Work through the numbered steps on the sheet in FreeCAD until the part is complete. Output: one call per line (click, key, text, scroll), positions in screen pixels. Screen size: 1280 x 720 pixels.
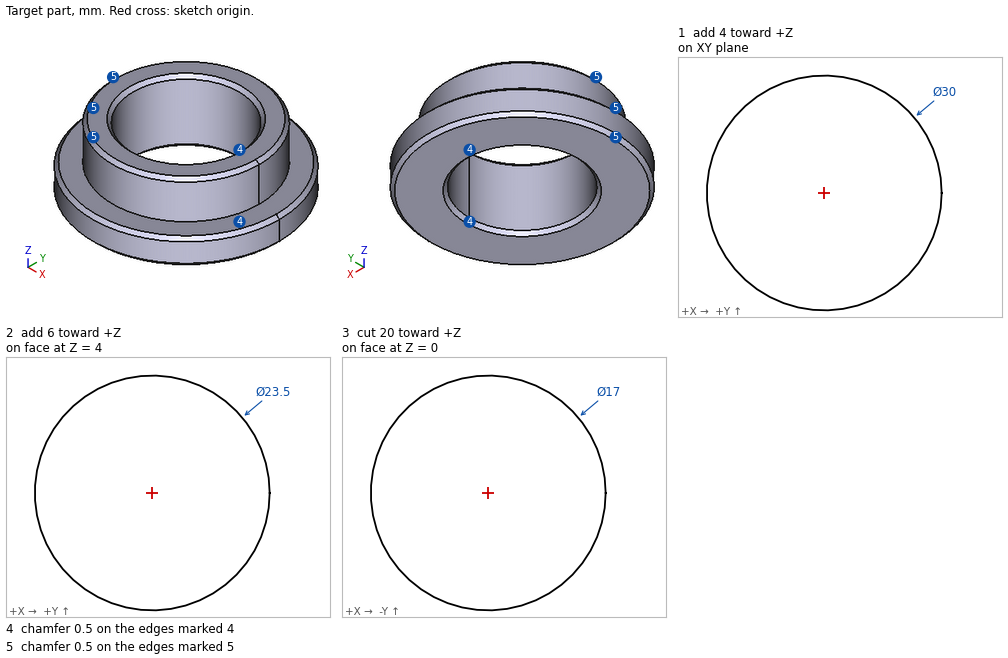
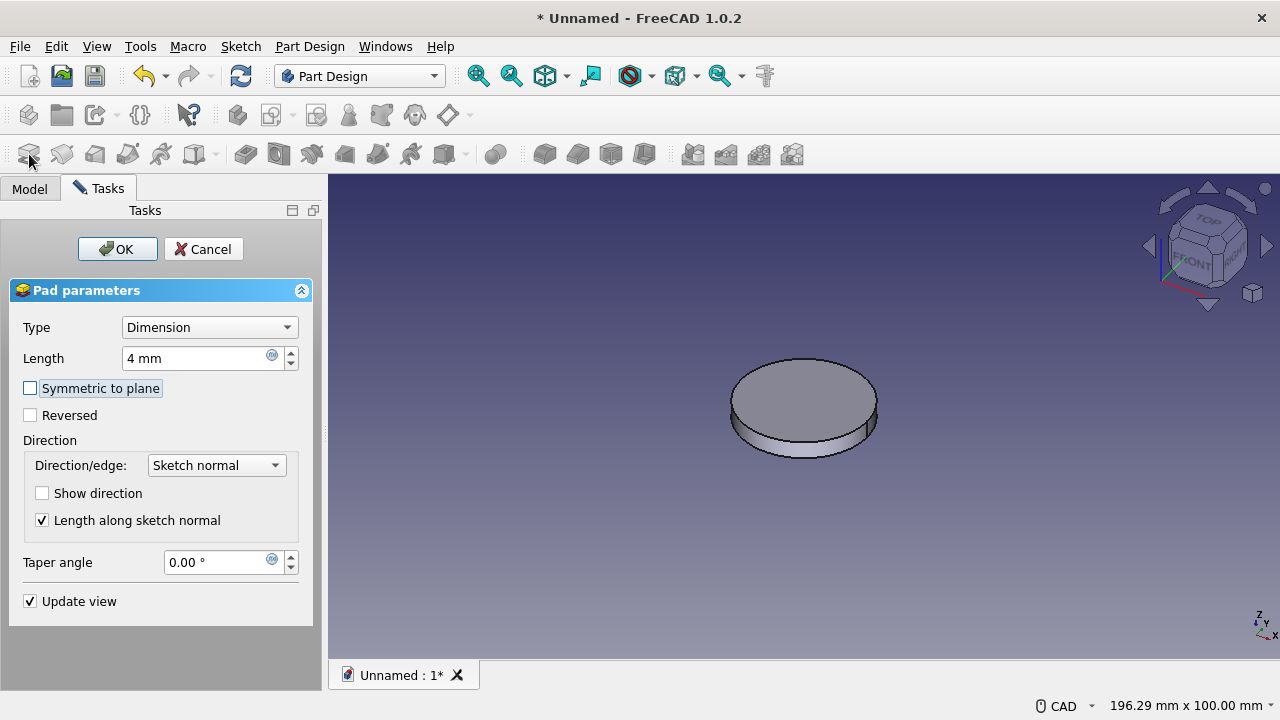
click(118, 249)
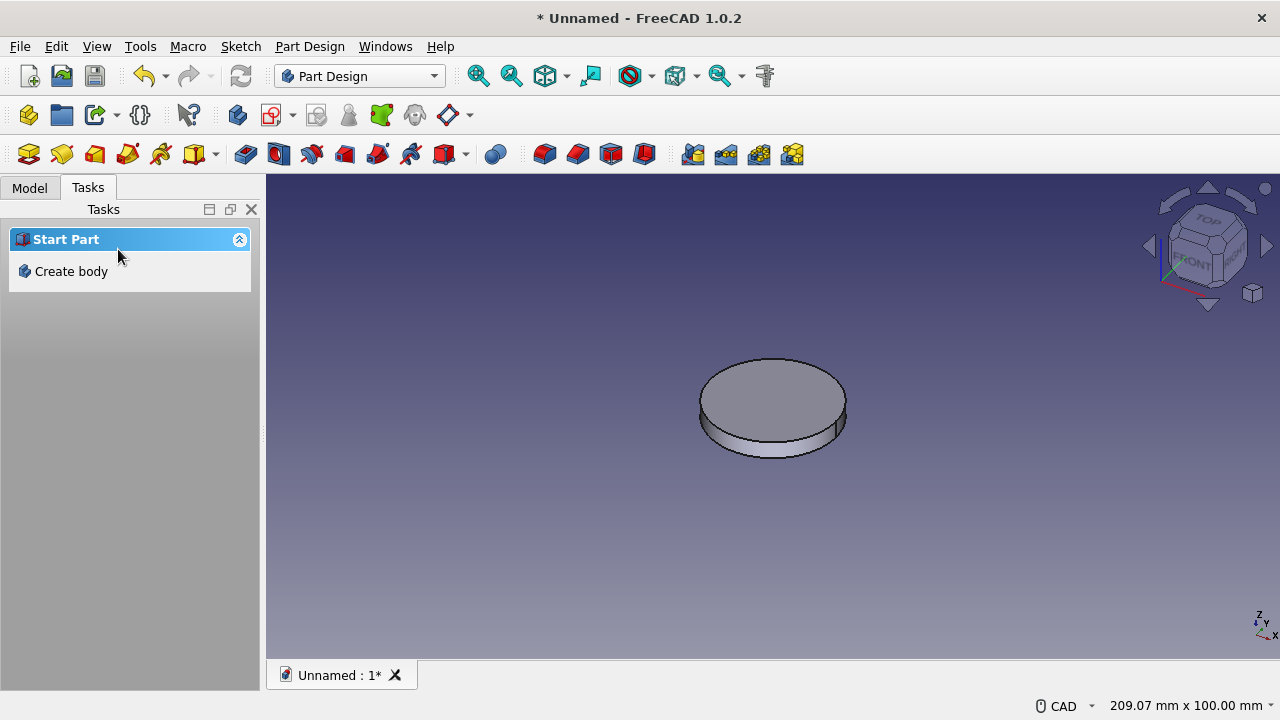
click(479, 76)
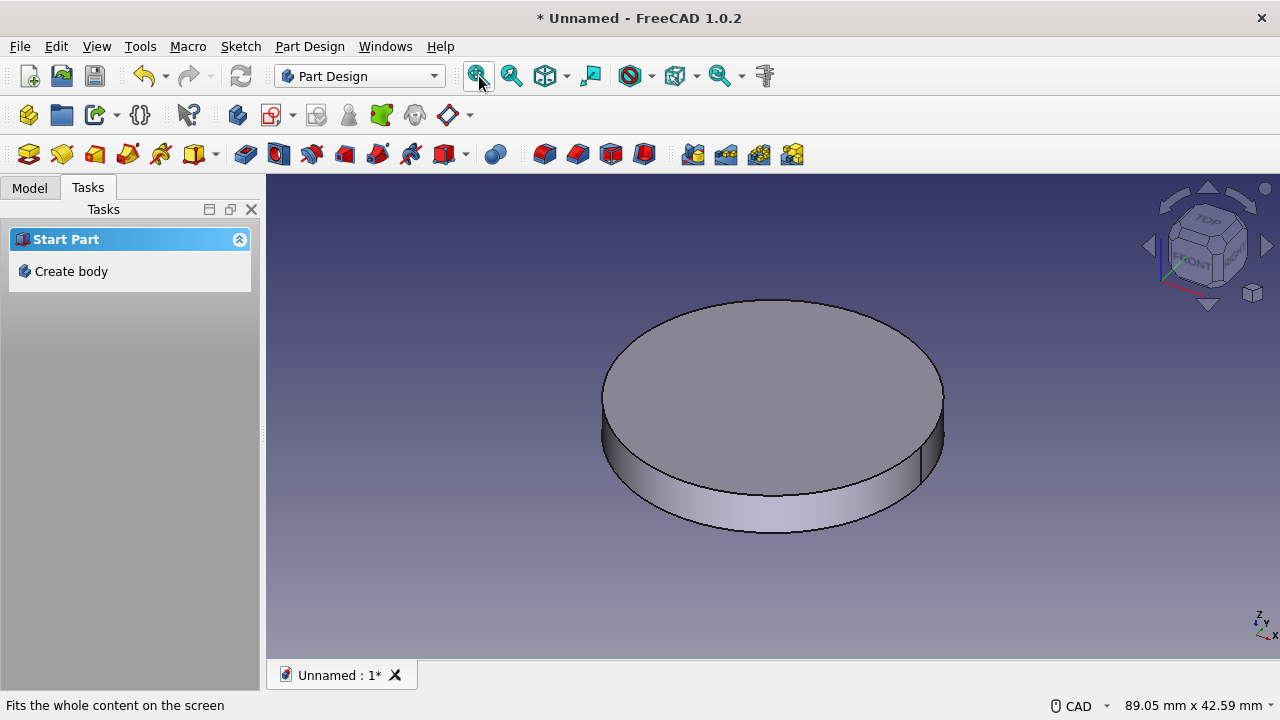
click(773, 397)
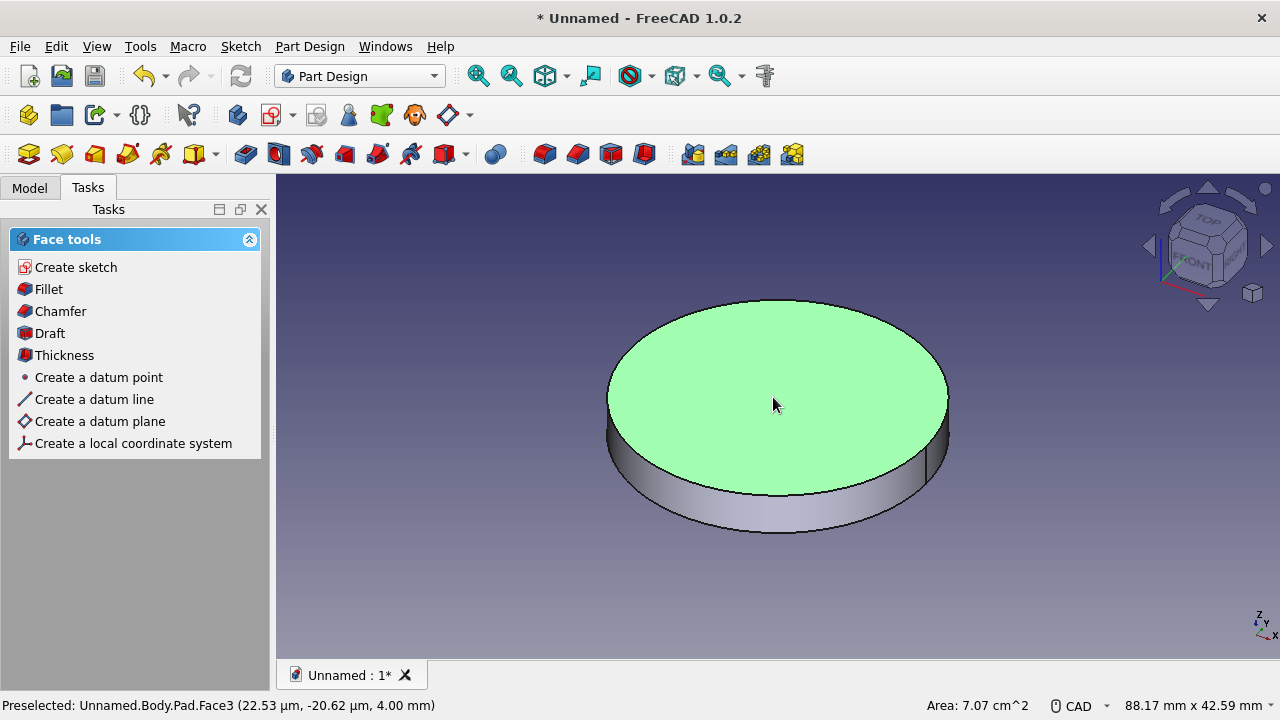
click(270, 116)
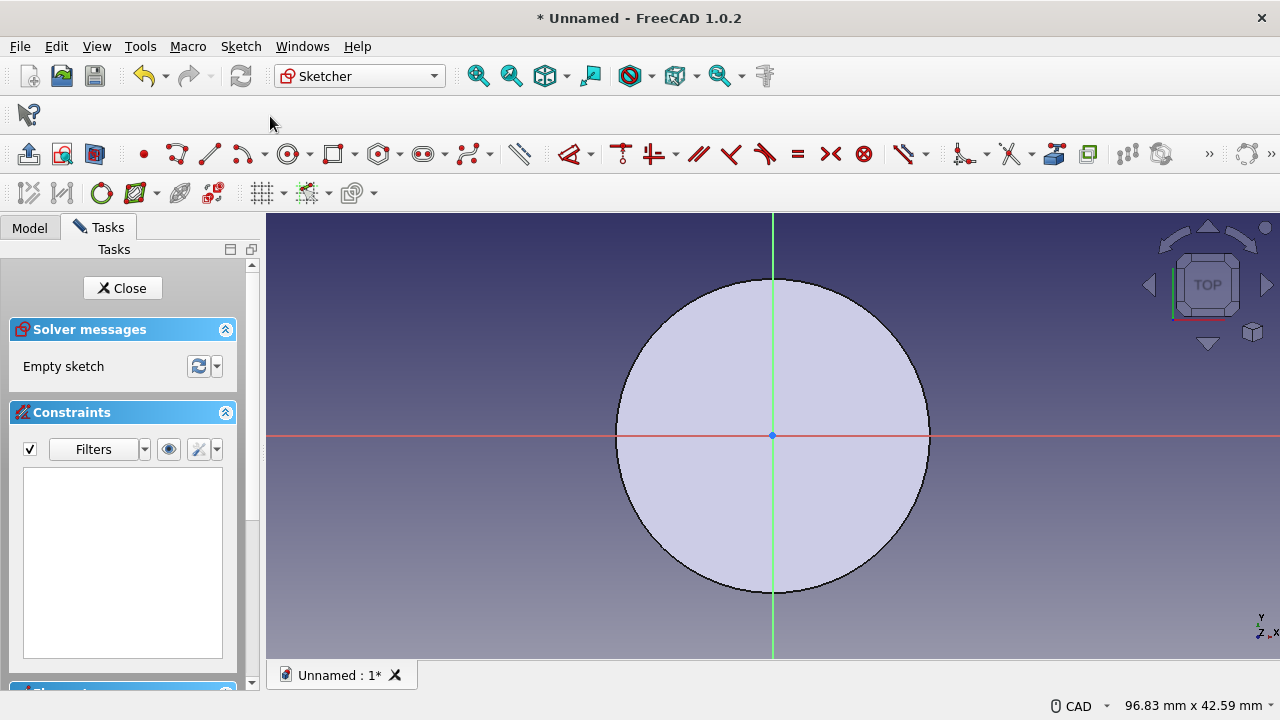
click(288, 154)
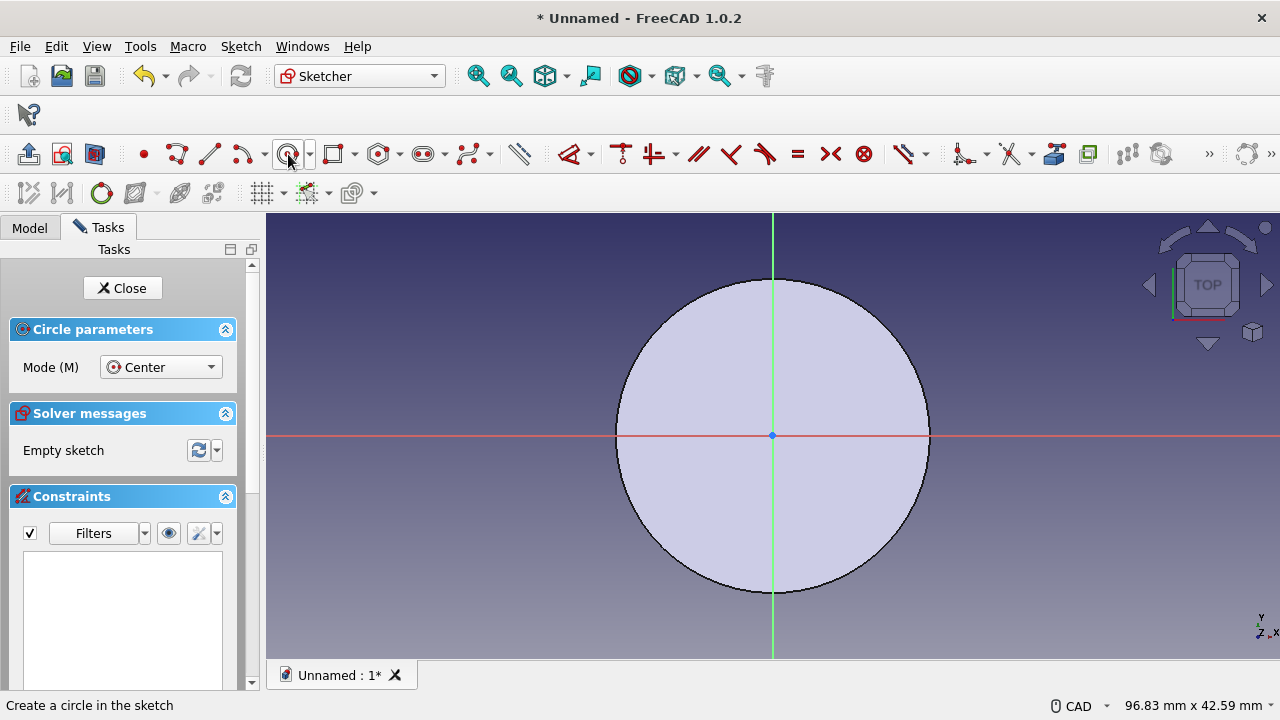
click(773, 436)
move(860, 349)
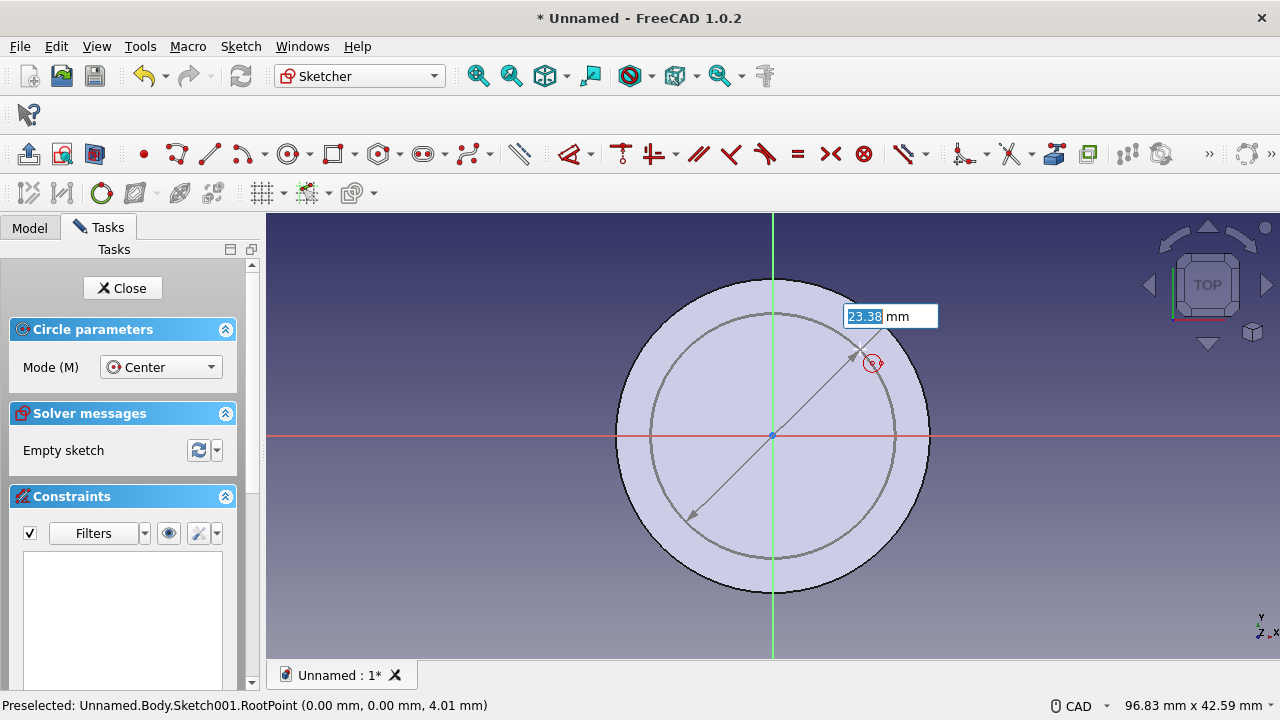
text(23.5)
key(Return)
key(Escape)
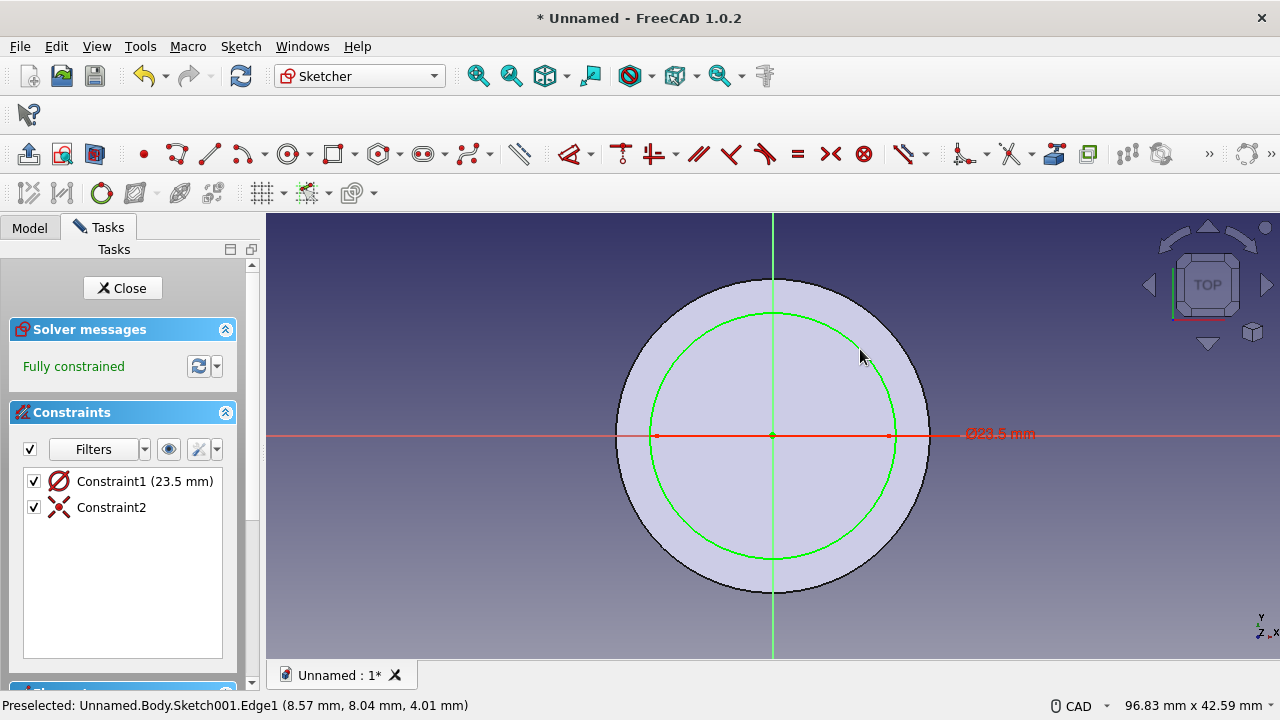
click(123, 288)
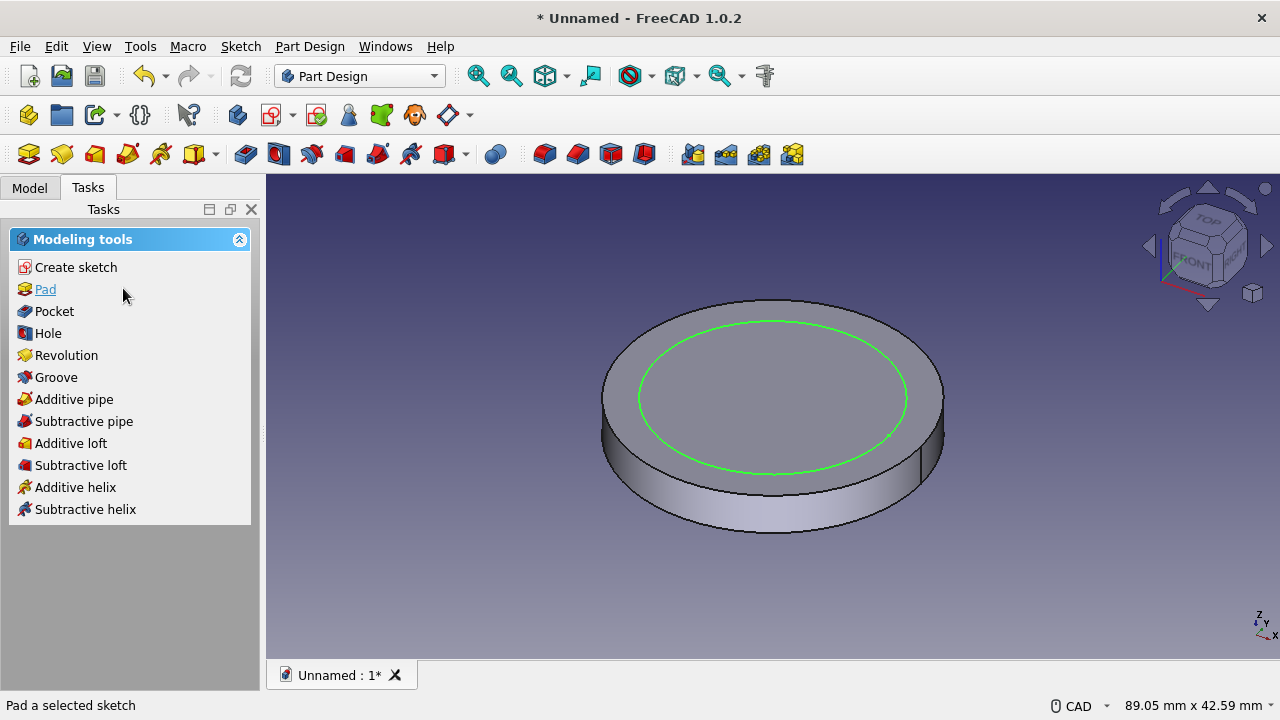
click(29, 154)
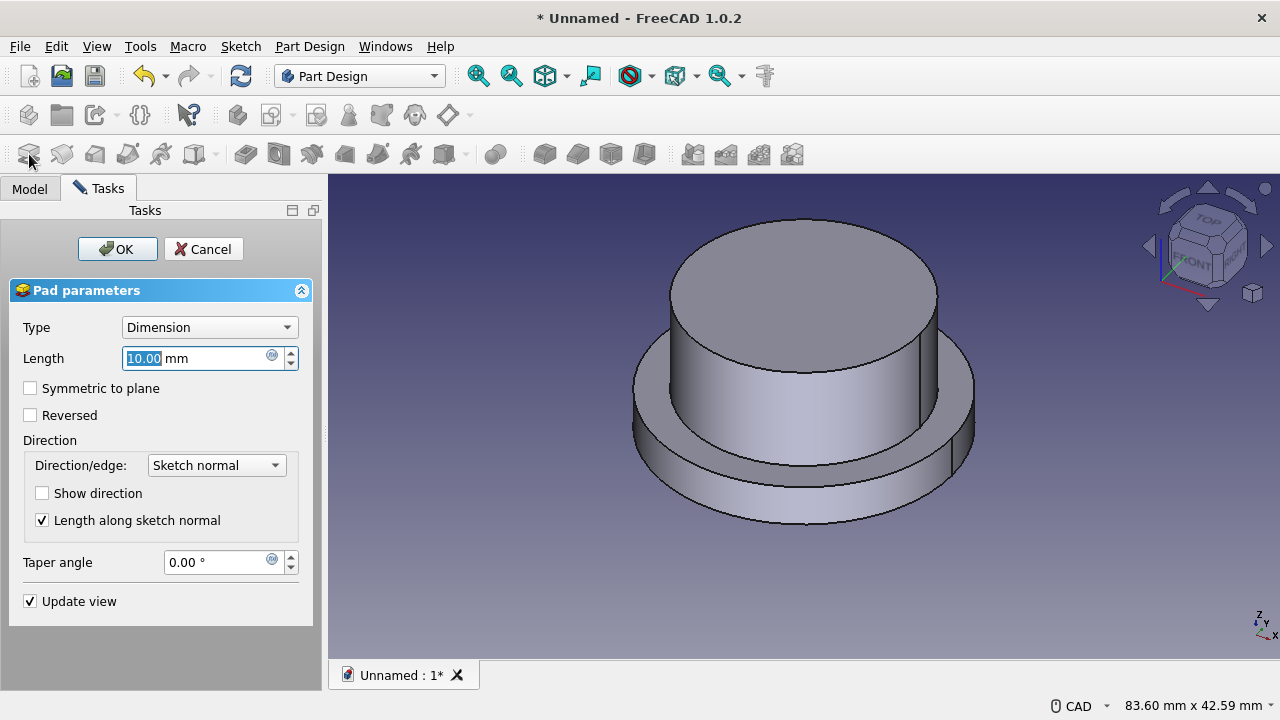
text(6)
key(Tab)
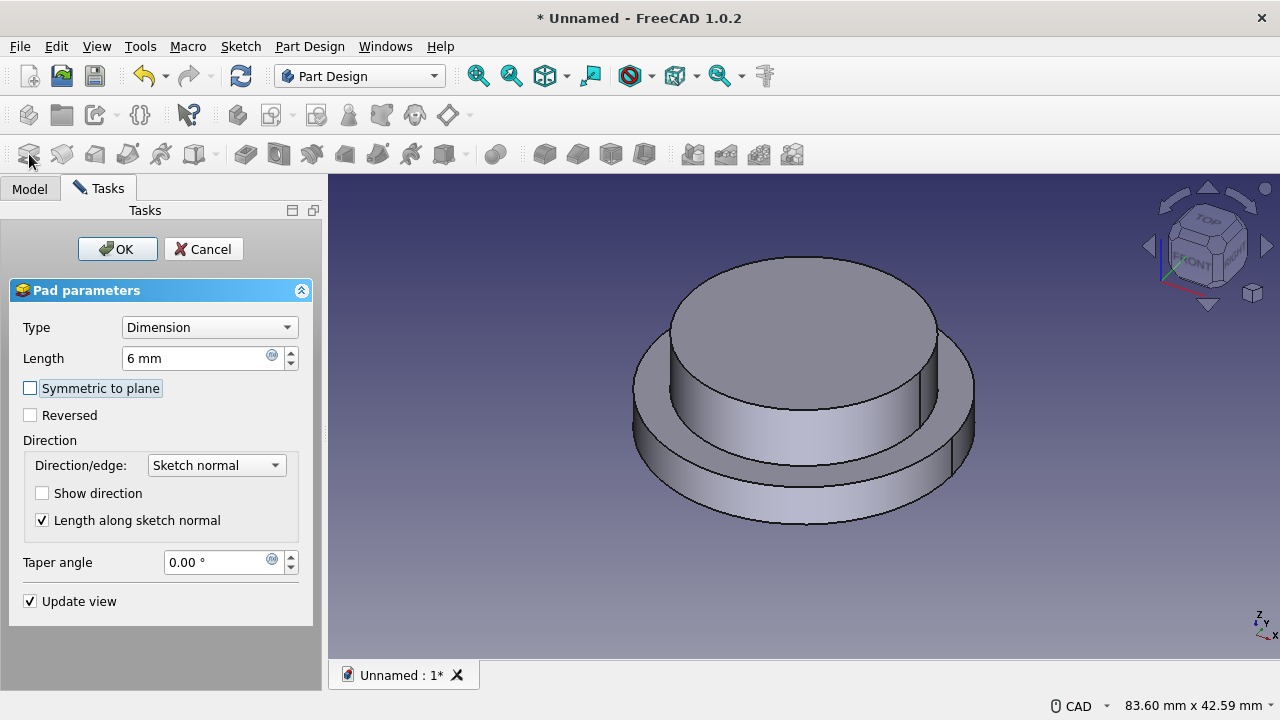
click(118, 249)